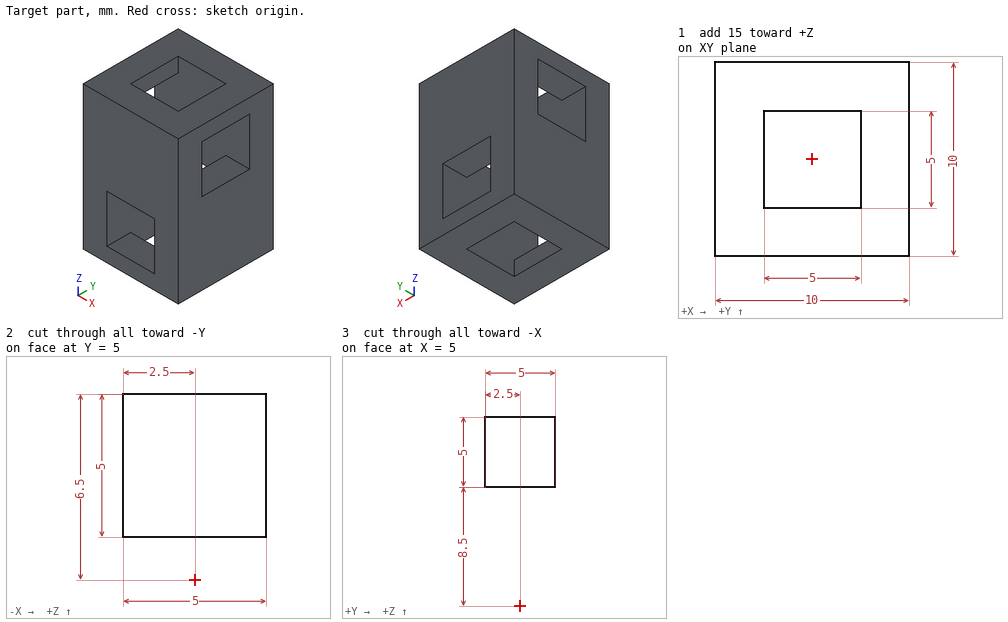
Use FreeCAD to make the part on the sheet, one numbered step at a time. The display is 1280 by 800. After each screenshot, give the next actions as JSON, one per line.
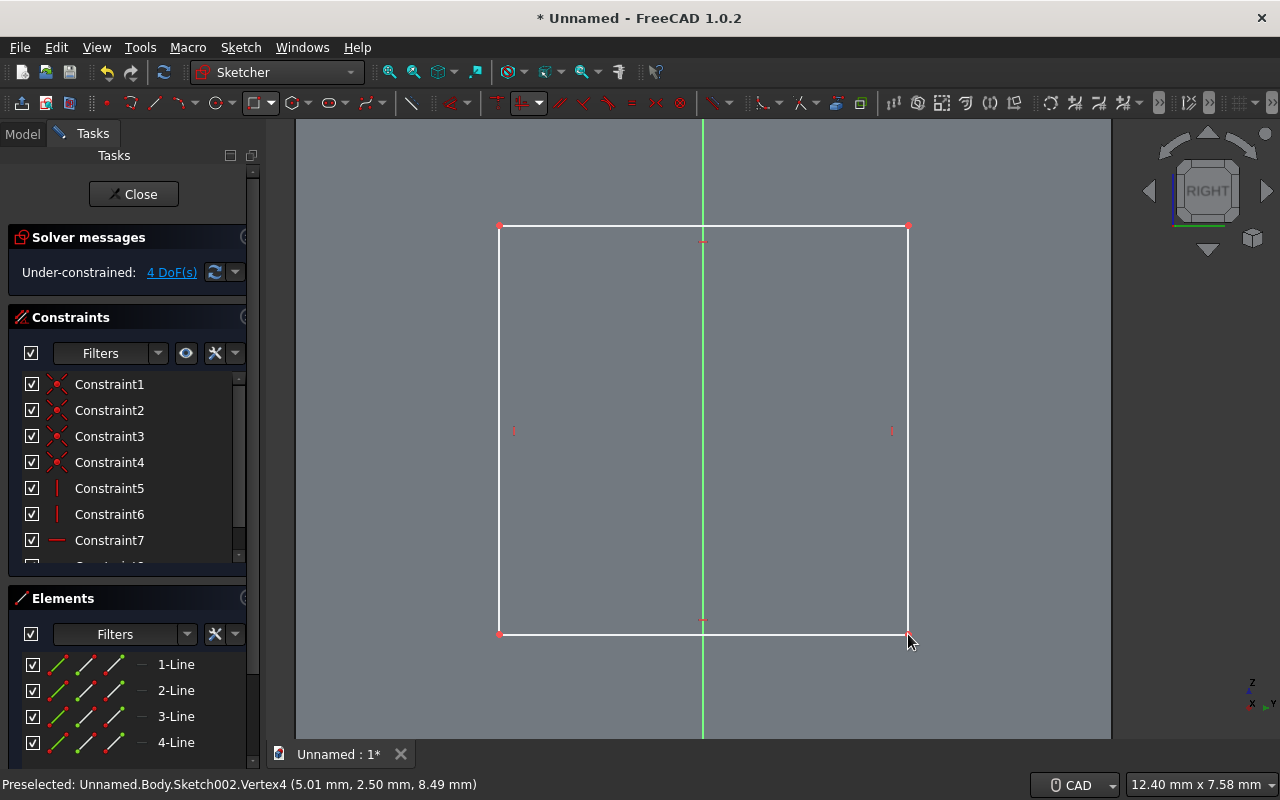
{"action": "left_click", "coordinate": [450, 104]}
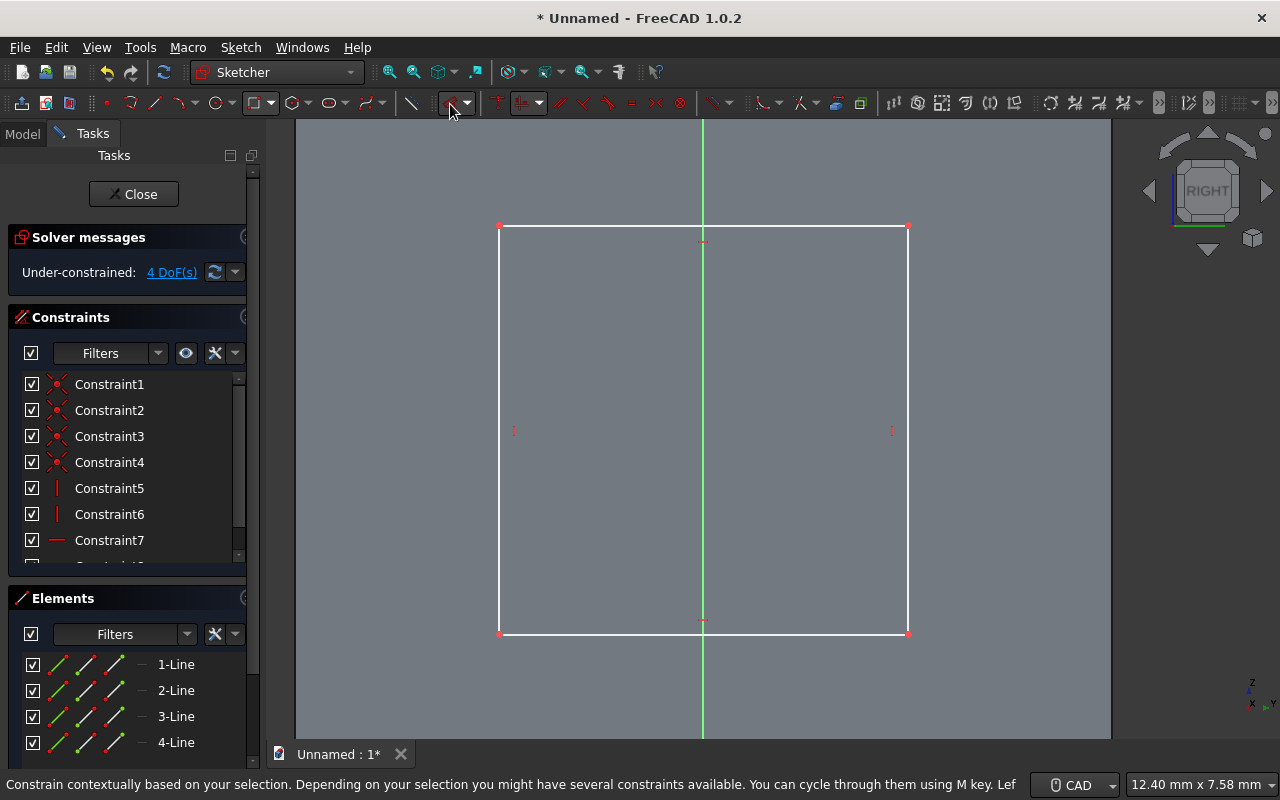
{"action": "left_click", "coordinate": [499, 349]}
{"action": "left_click", "coordinate": [465, 430]}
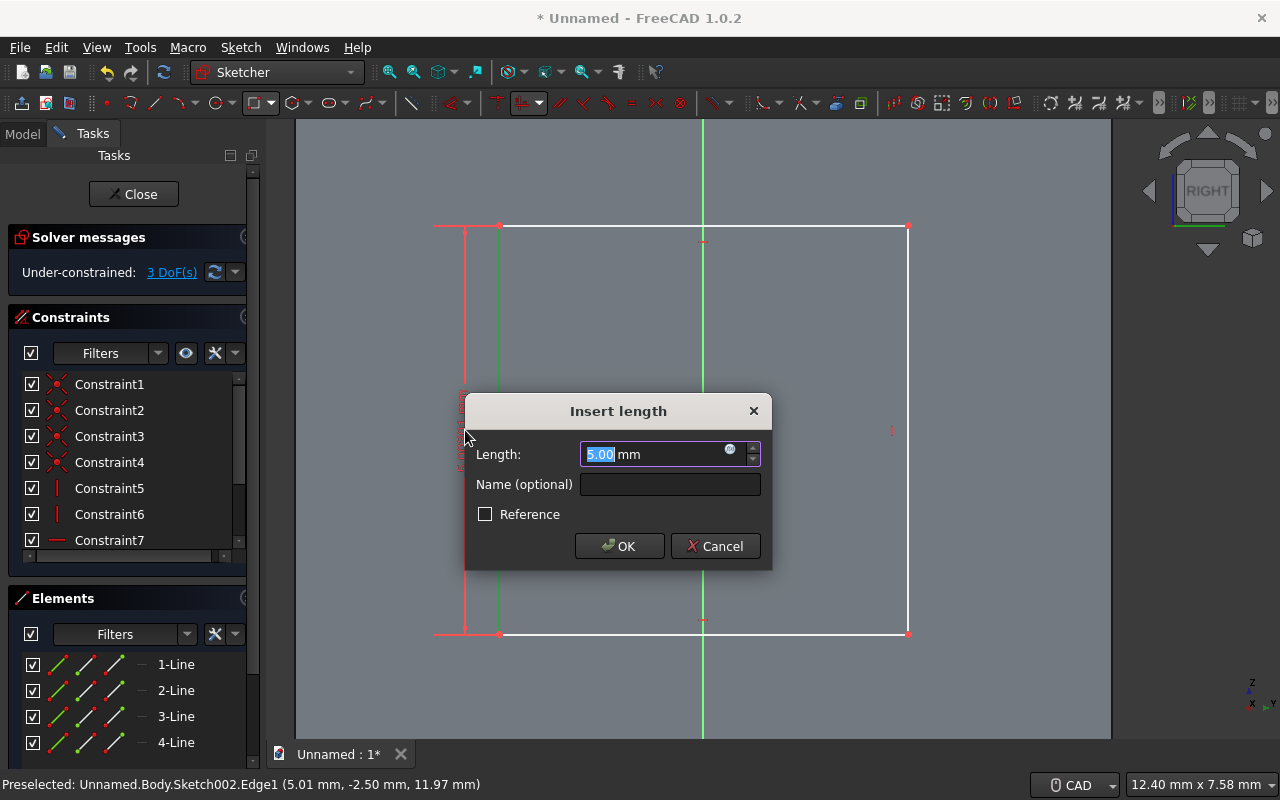
{"action": "type", "text": "5"}
{"action": "key", "text": "Return"}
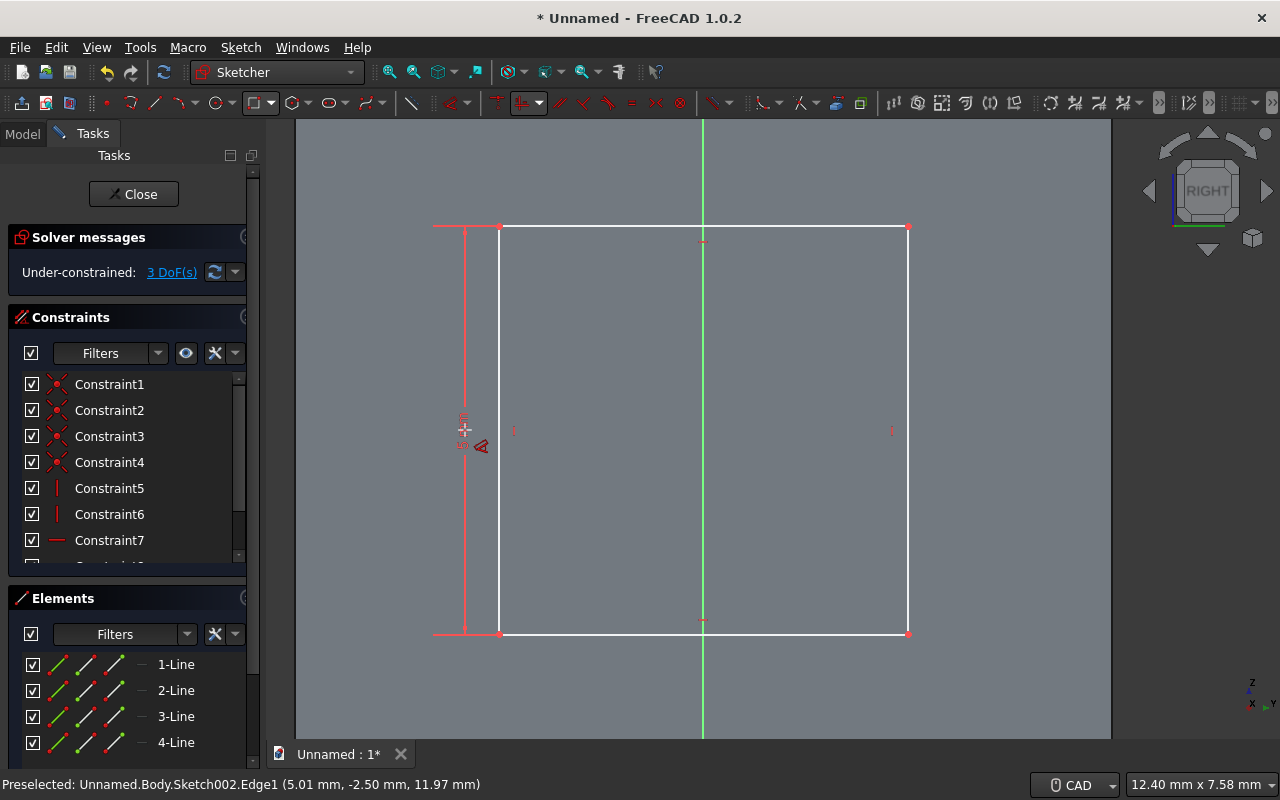
{"action": "left_click", "coordinate": [622, 635]}
{"action": "left_click", "coordinate": [609, 669]}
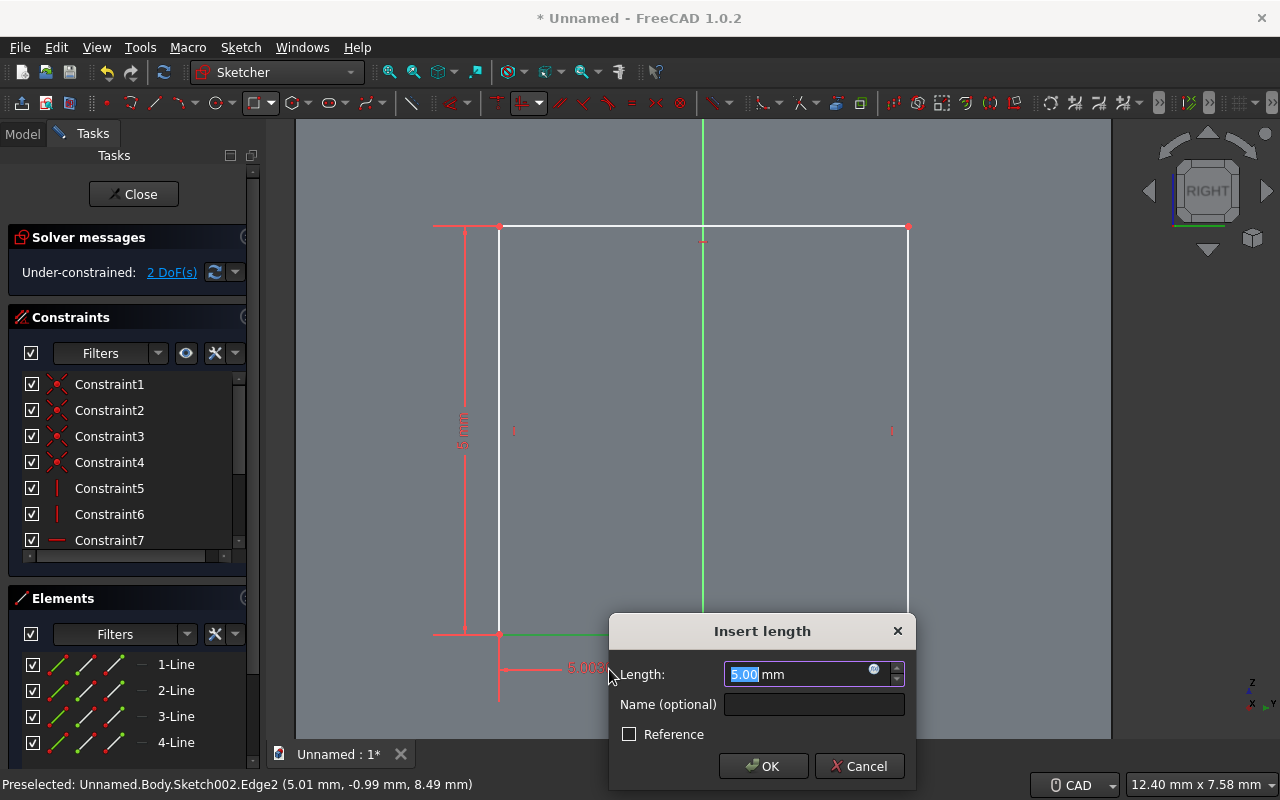
{"action": "type", "text": "5"}
{"action": "key", "text": "Return"}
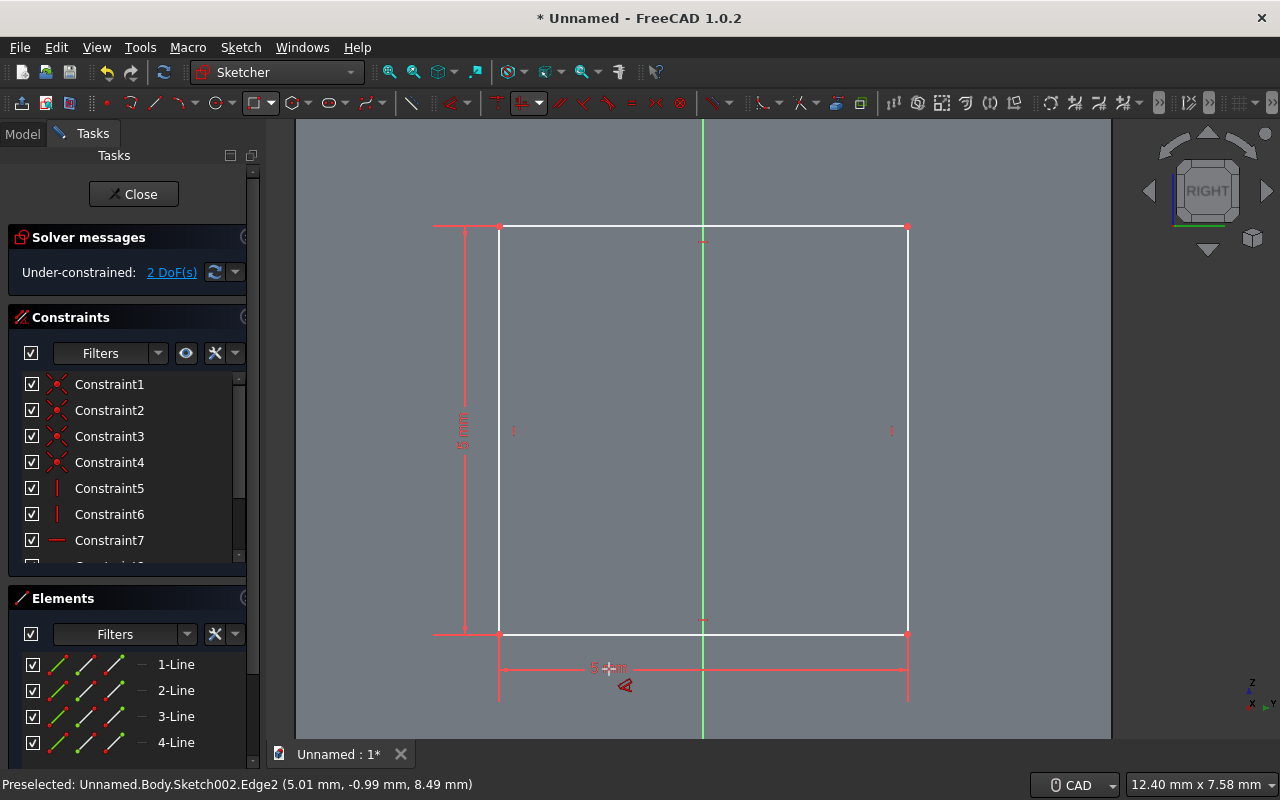
{"action": "left_click", "coordinate": [499, 226]}
{"action": "left_click", "coordinate": [601, 192]}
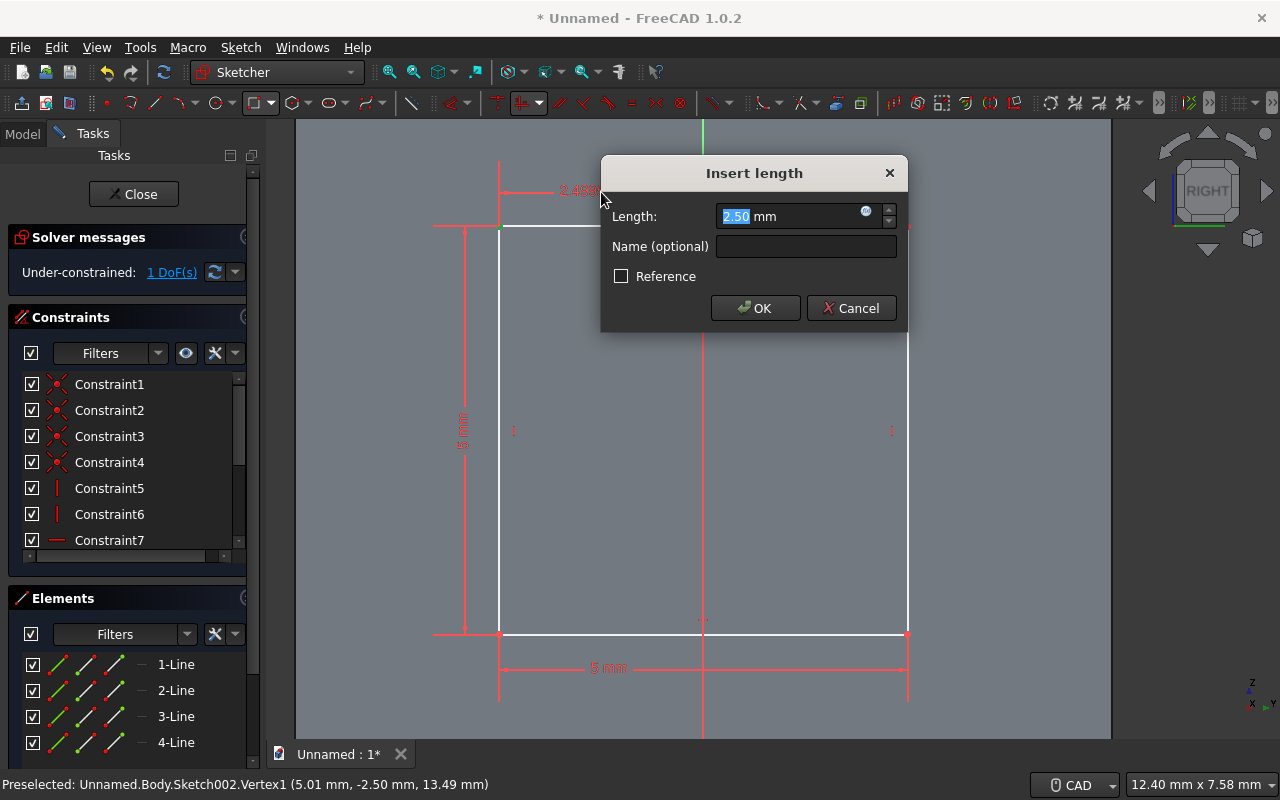
{"action": "type", "text": "2.5"}
{"action": "key", "text": "Return"}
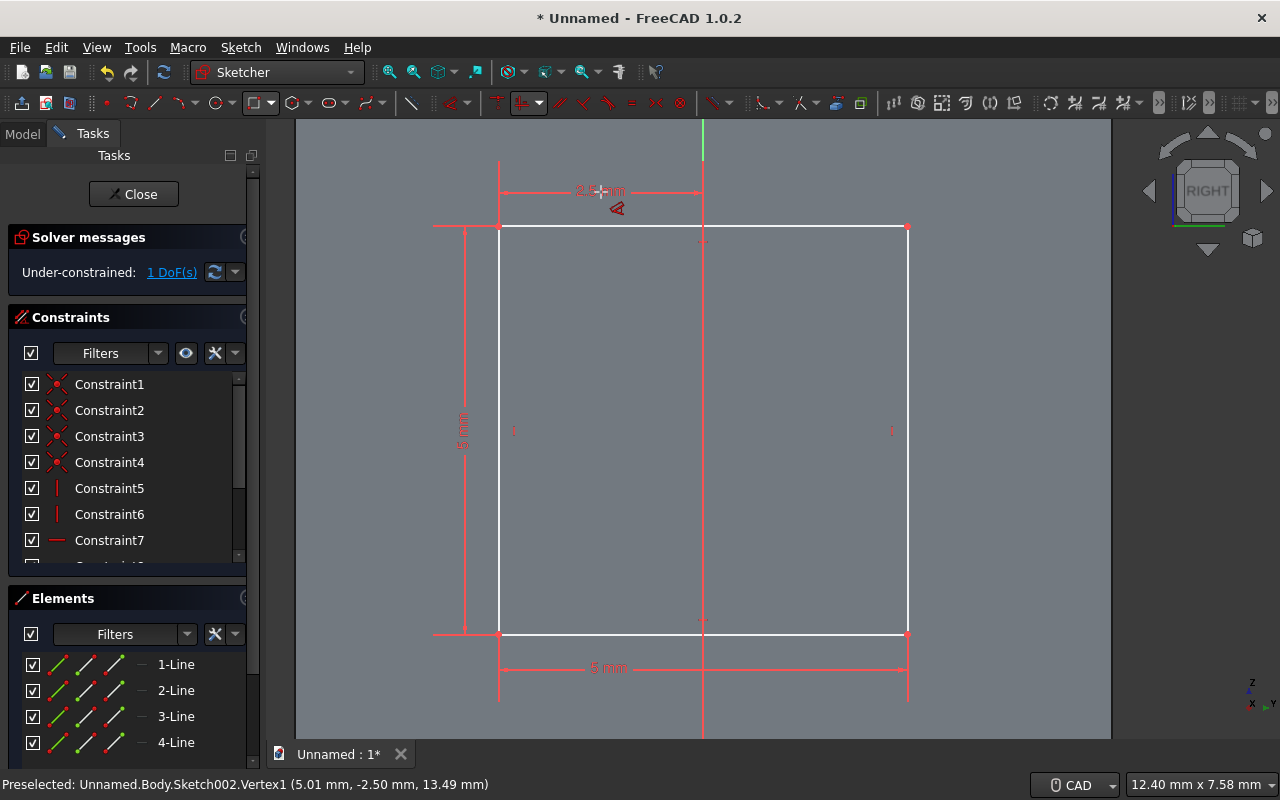
{"action": "left_click", "coordinate": [499, 635]}
{"action": "left_click", "coordinate": [465, 673]}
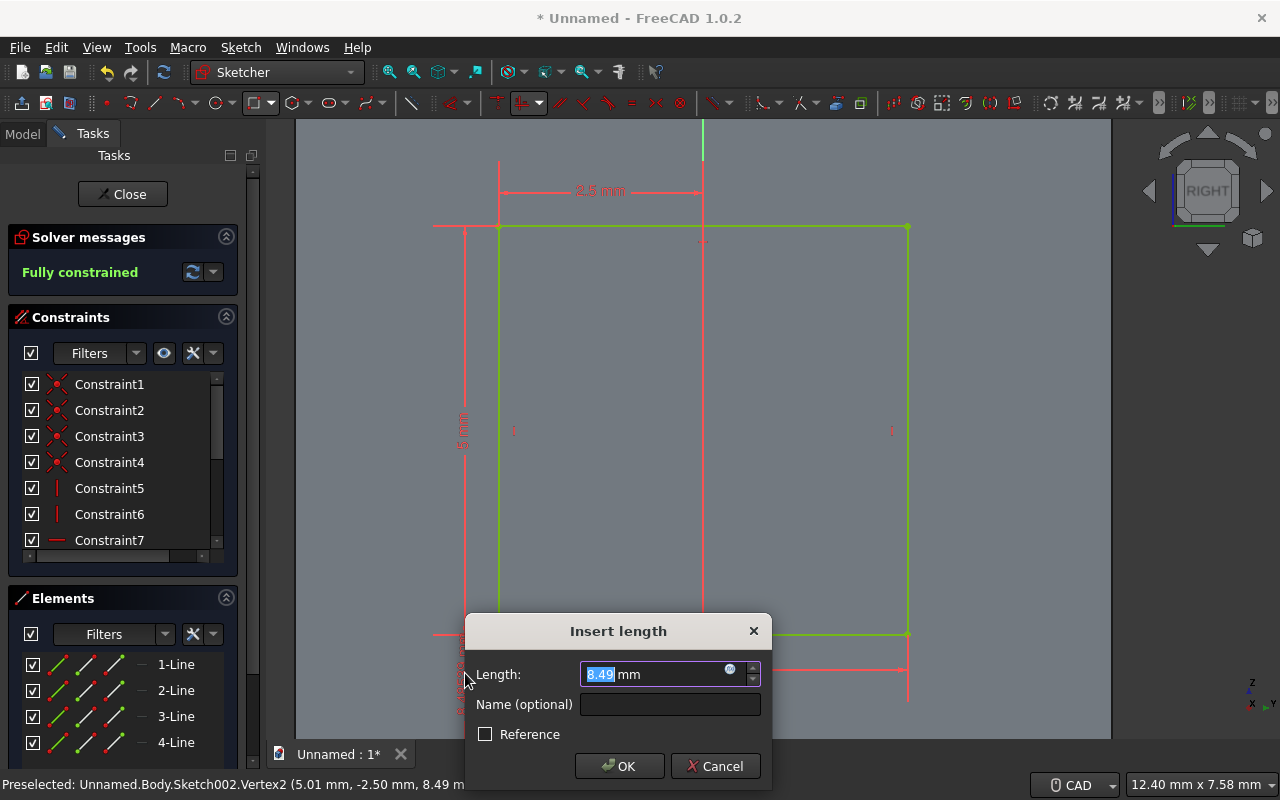
{"action": "type", "text": "8.5"}
{"action": "key", "text": "Return"}
{"action": "key", "text": "Escape"}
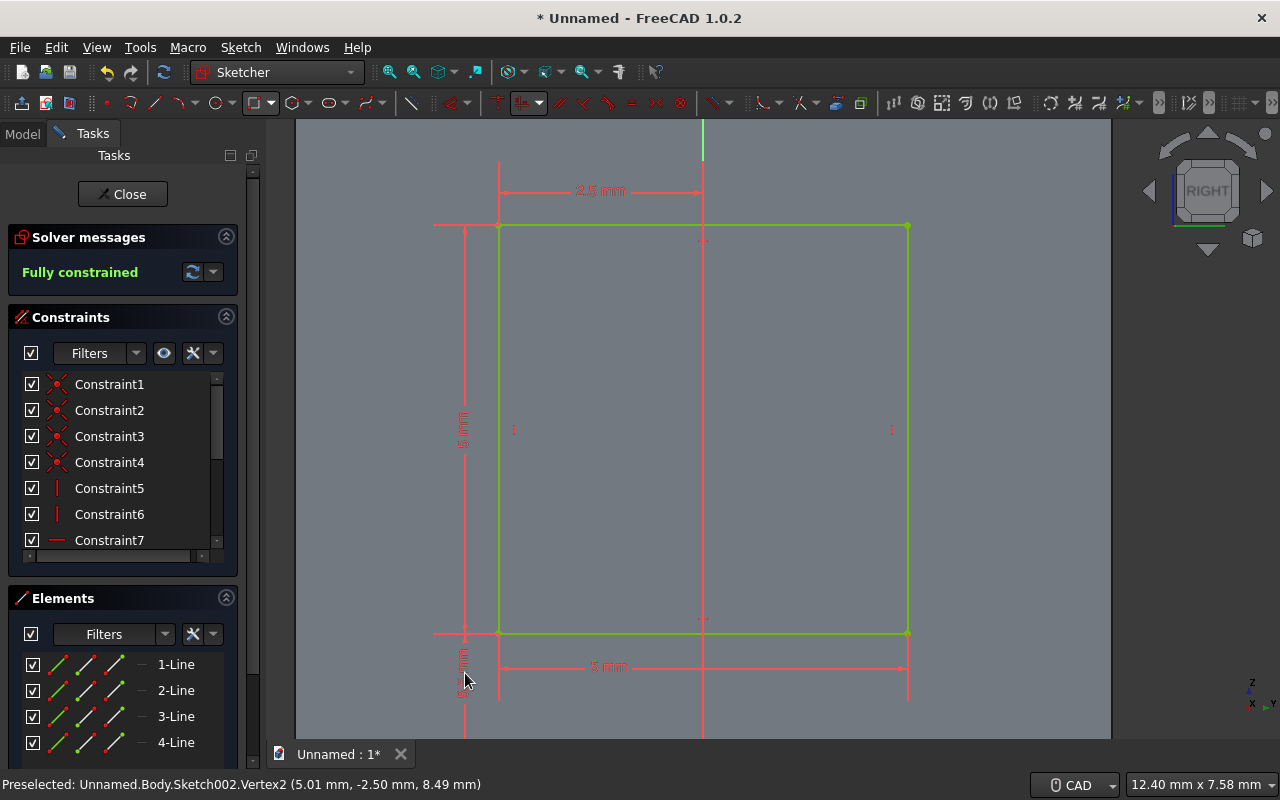
{"action": "left_click", "coordinate": [123, 194]}